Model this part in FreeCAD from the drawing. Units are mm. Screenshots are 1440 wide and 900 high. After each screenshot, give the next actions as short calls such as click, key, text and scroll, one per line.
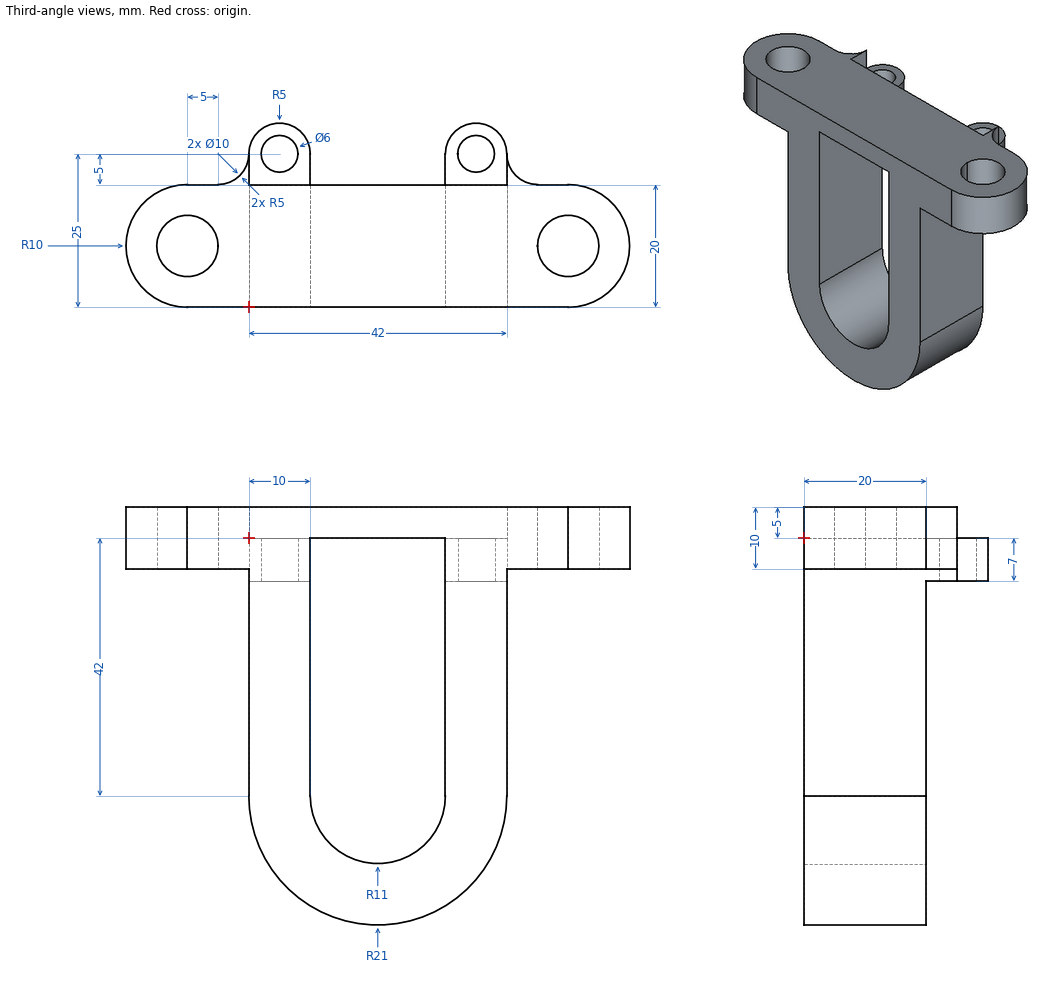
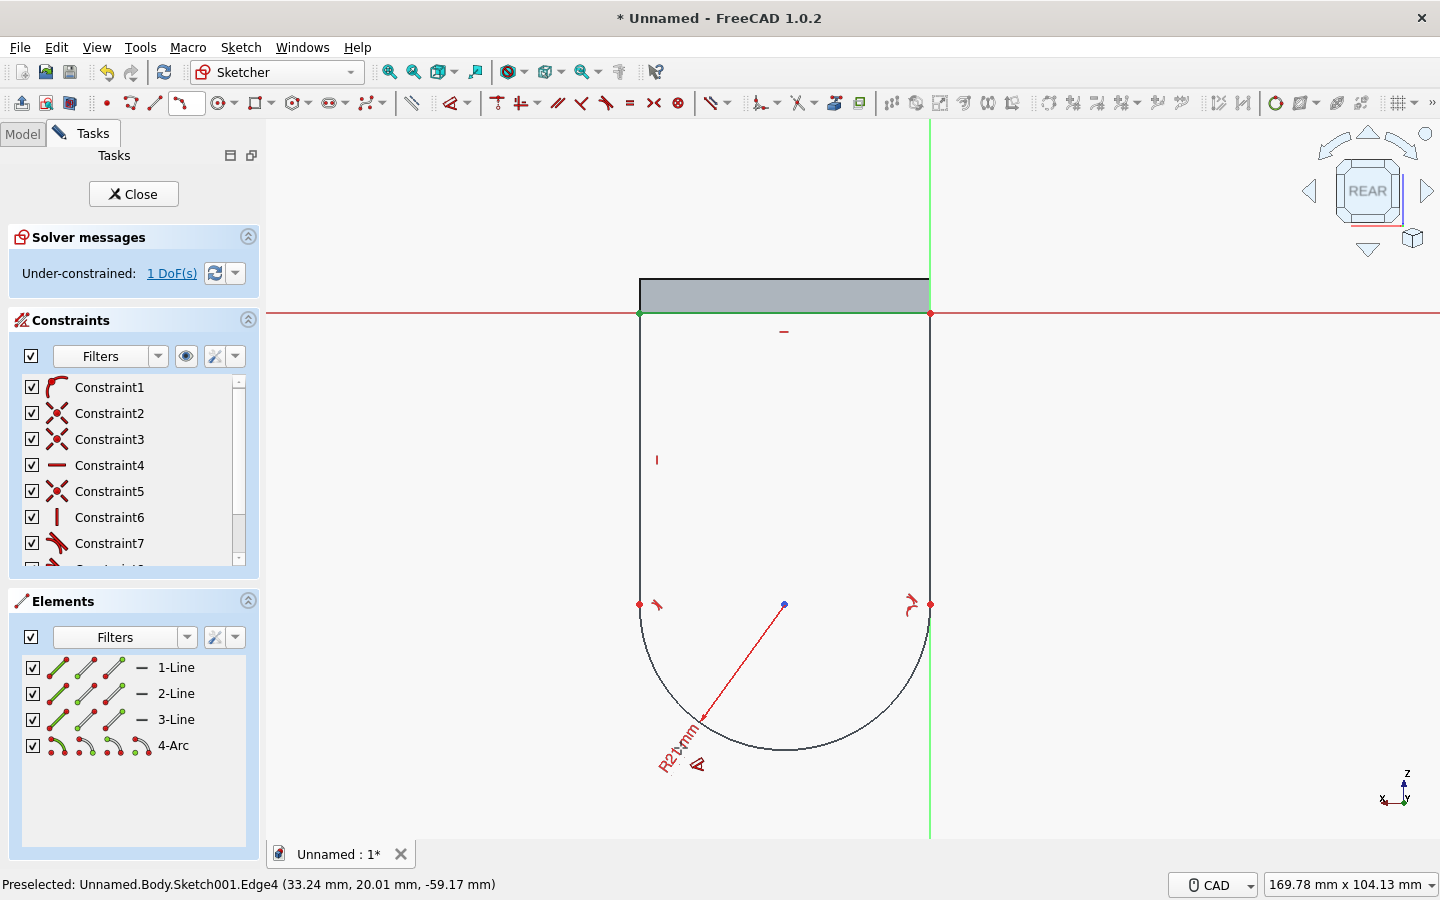
click(930, 517)
click(964, 459)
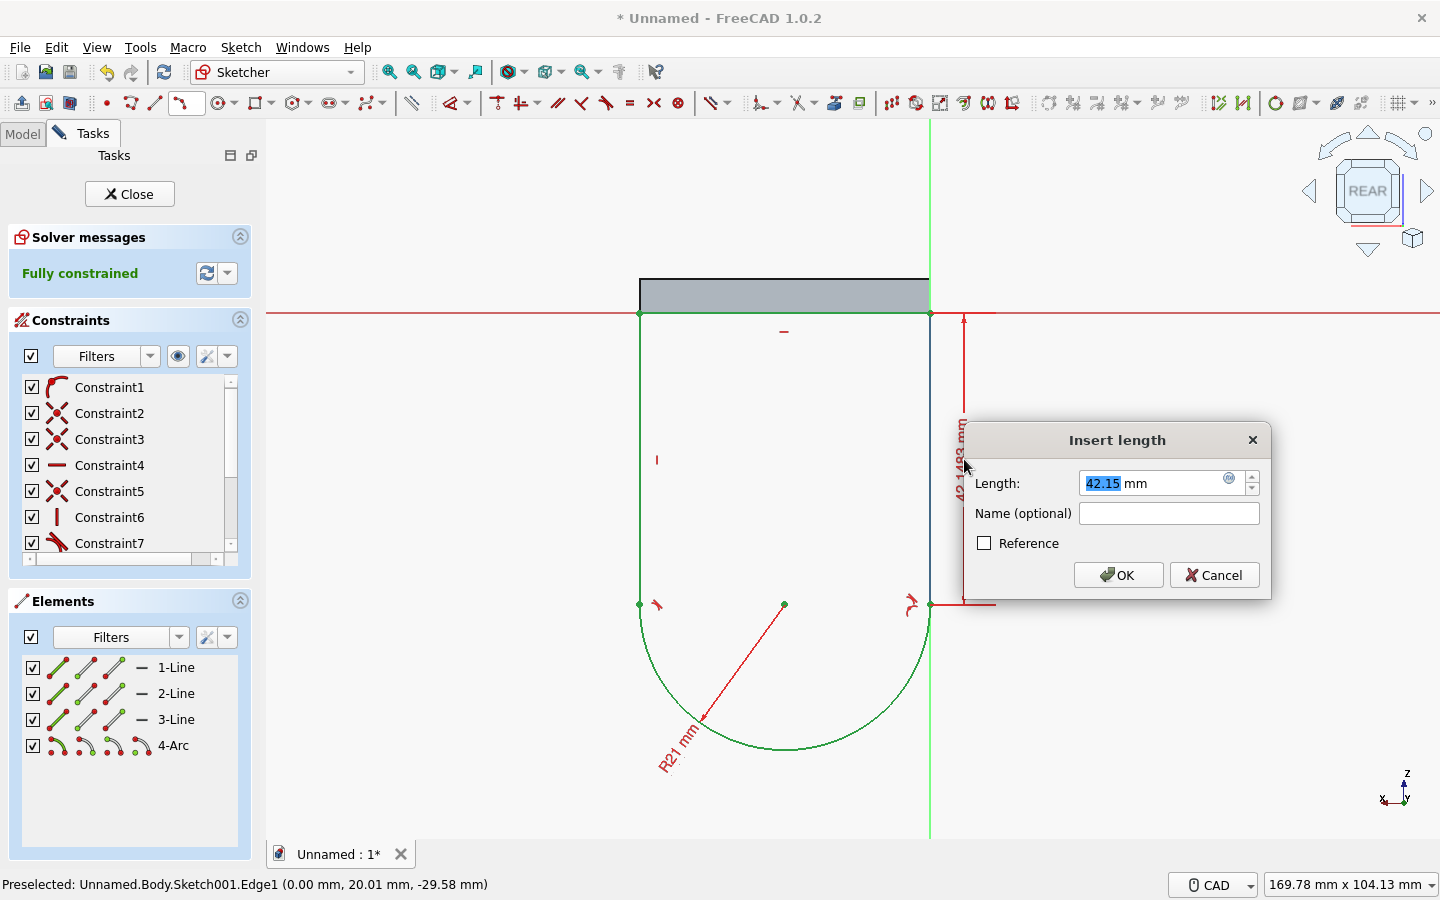
text(42)
key(Return)
key(Escape)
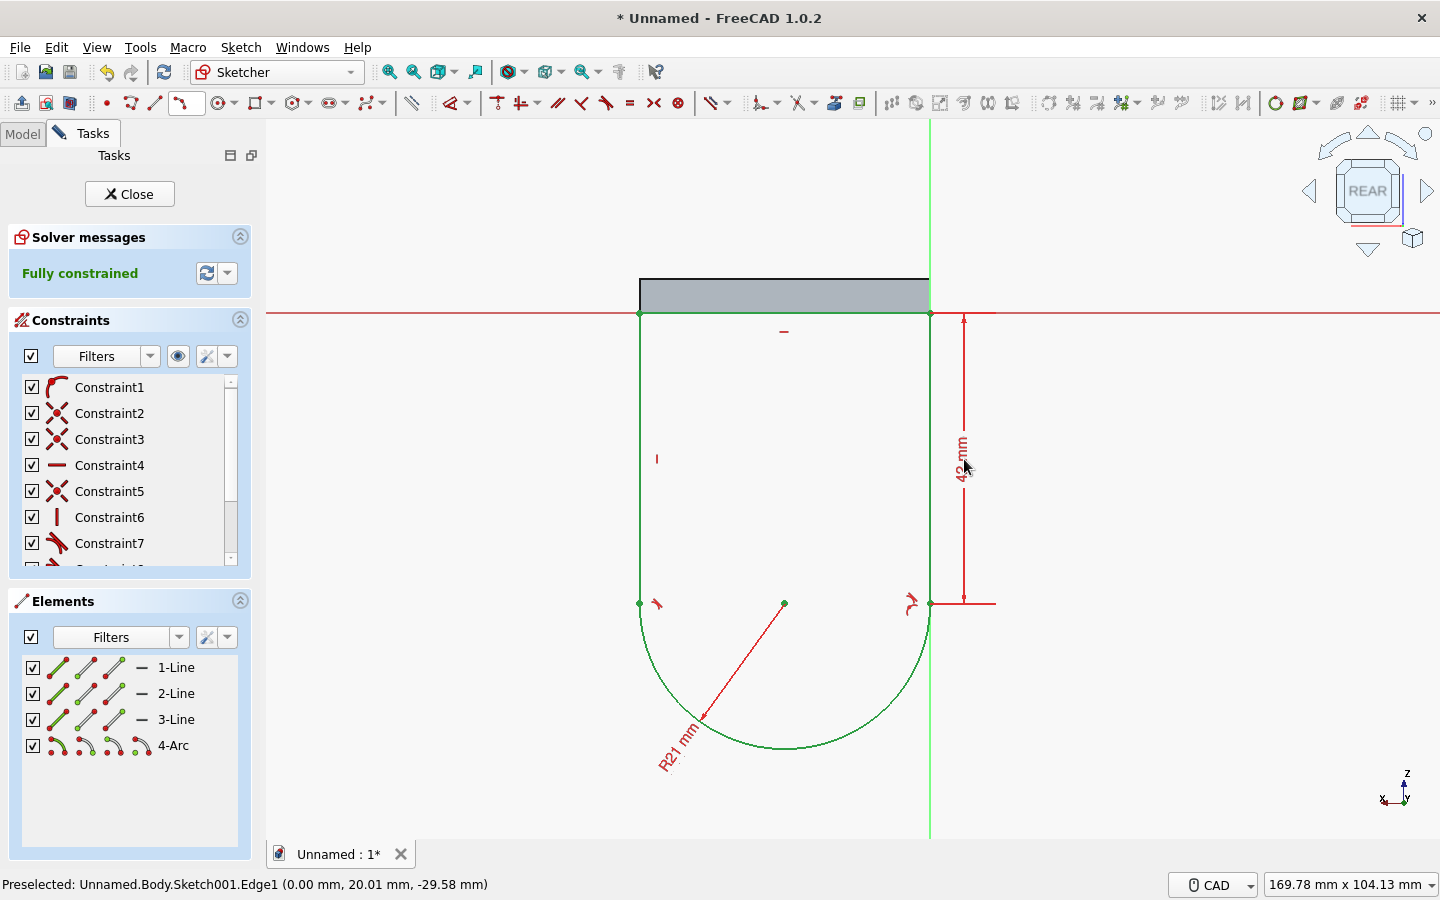
click(130, 194)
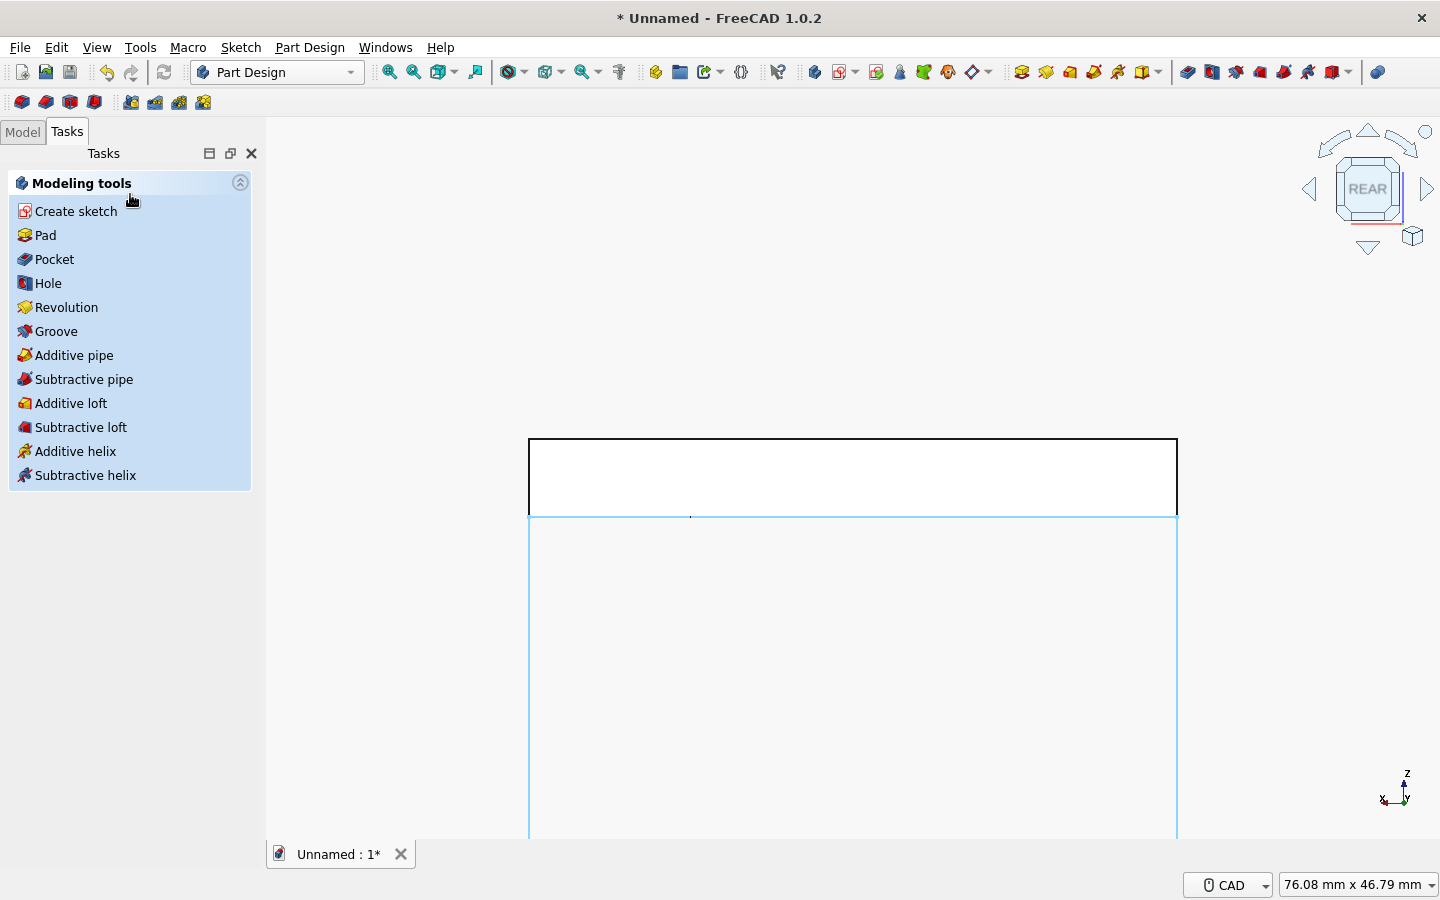
click(1022, 72)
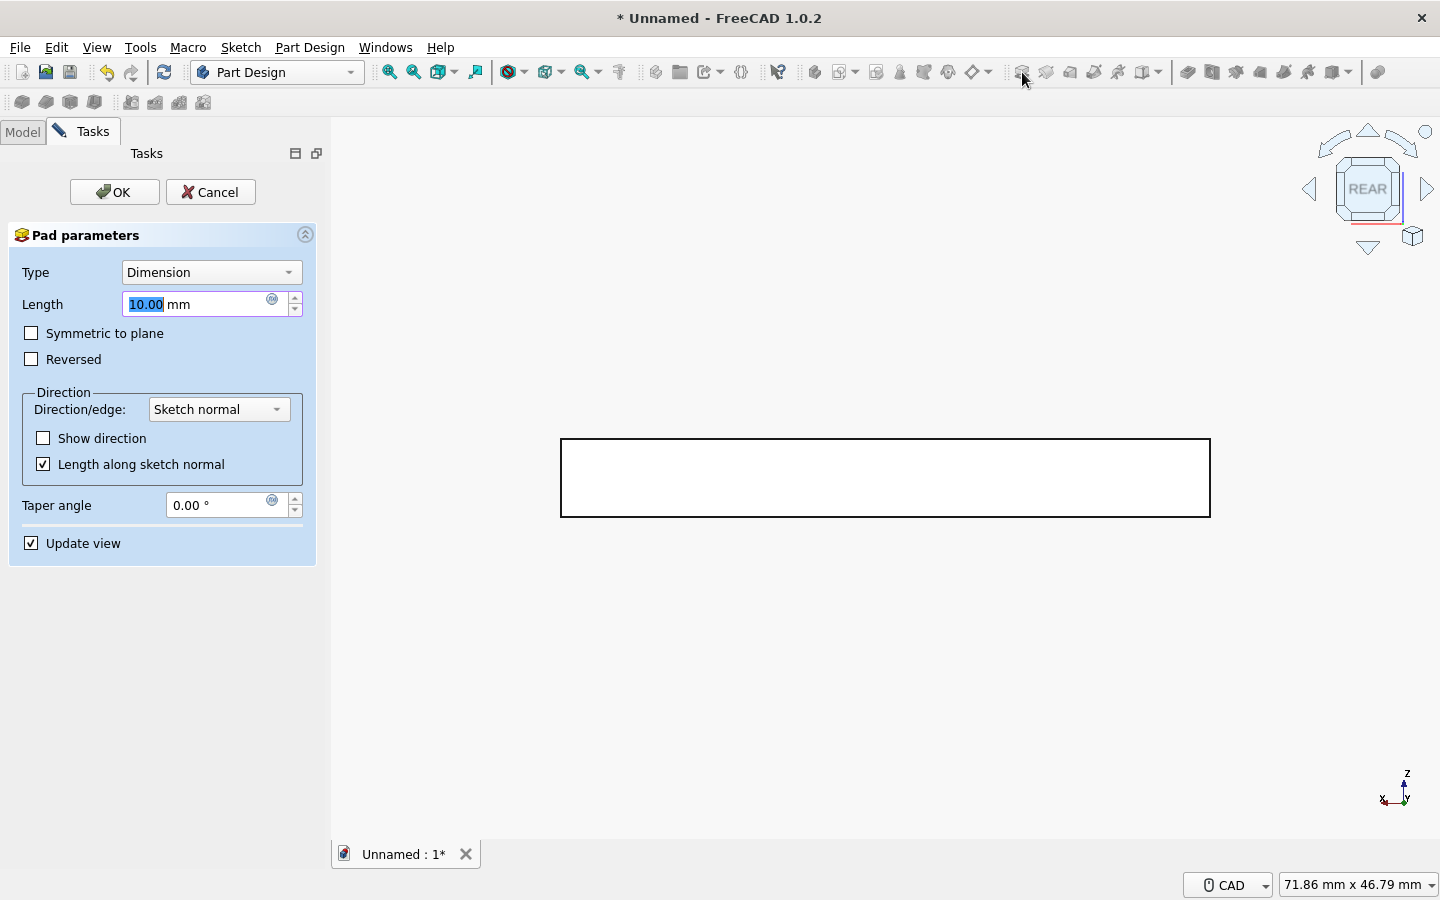
text(20)
key(Tab)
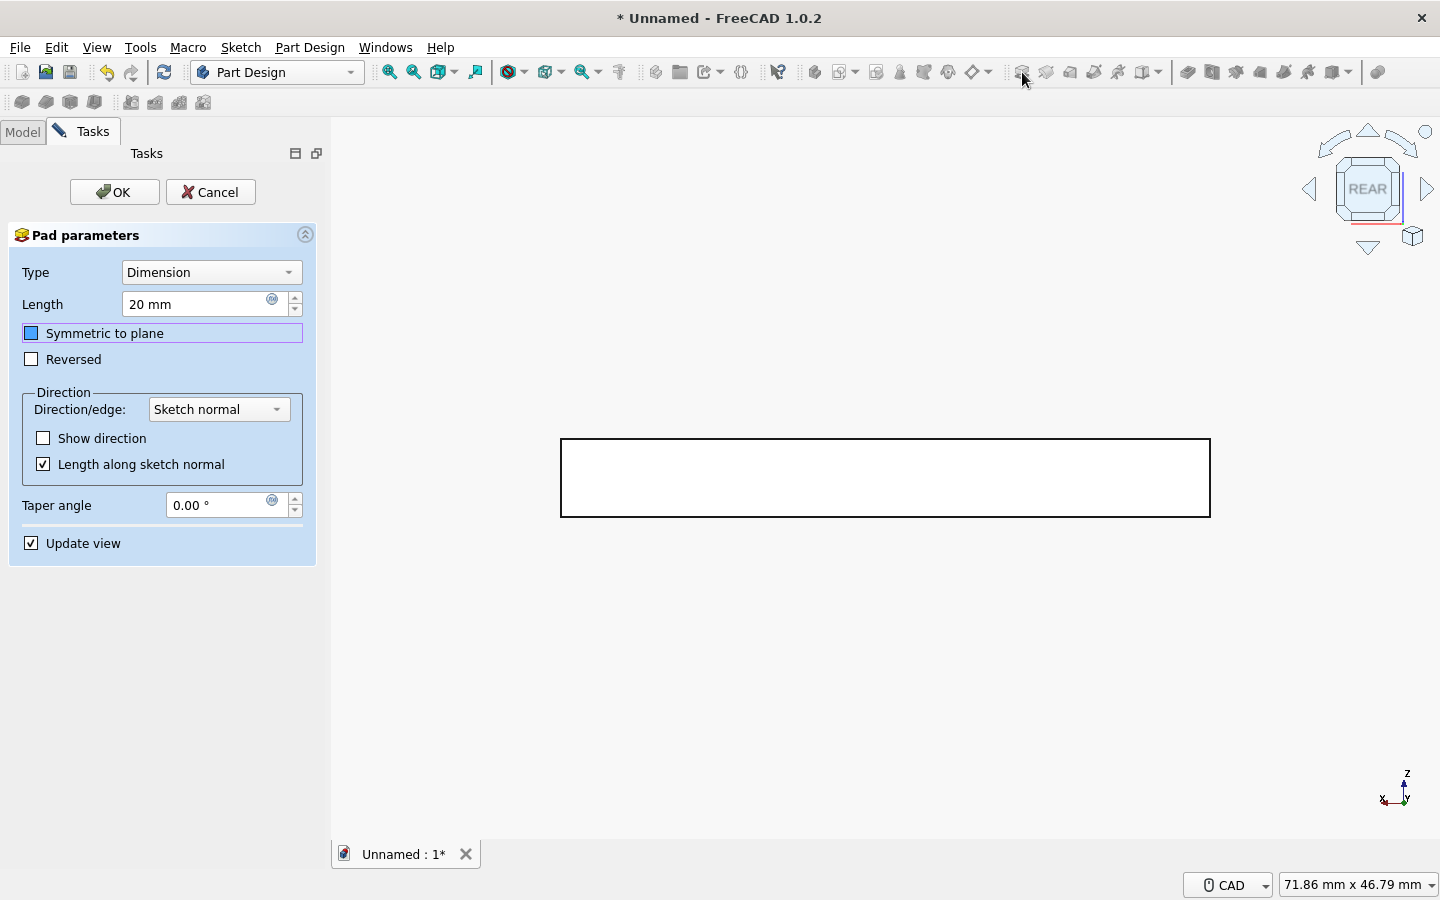
click(30, 359)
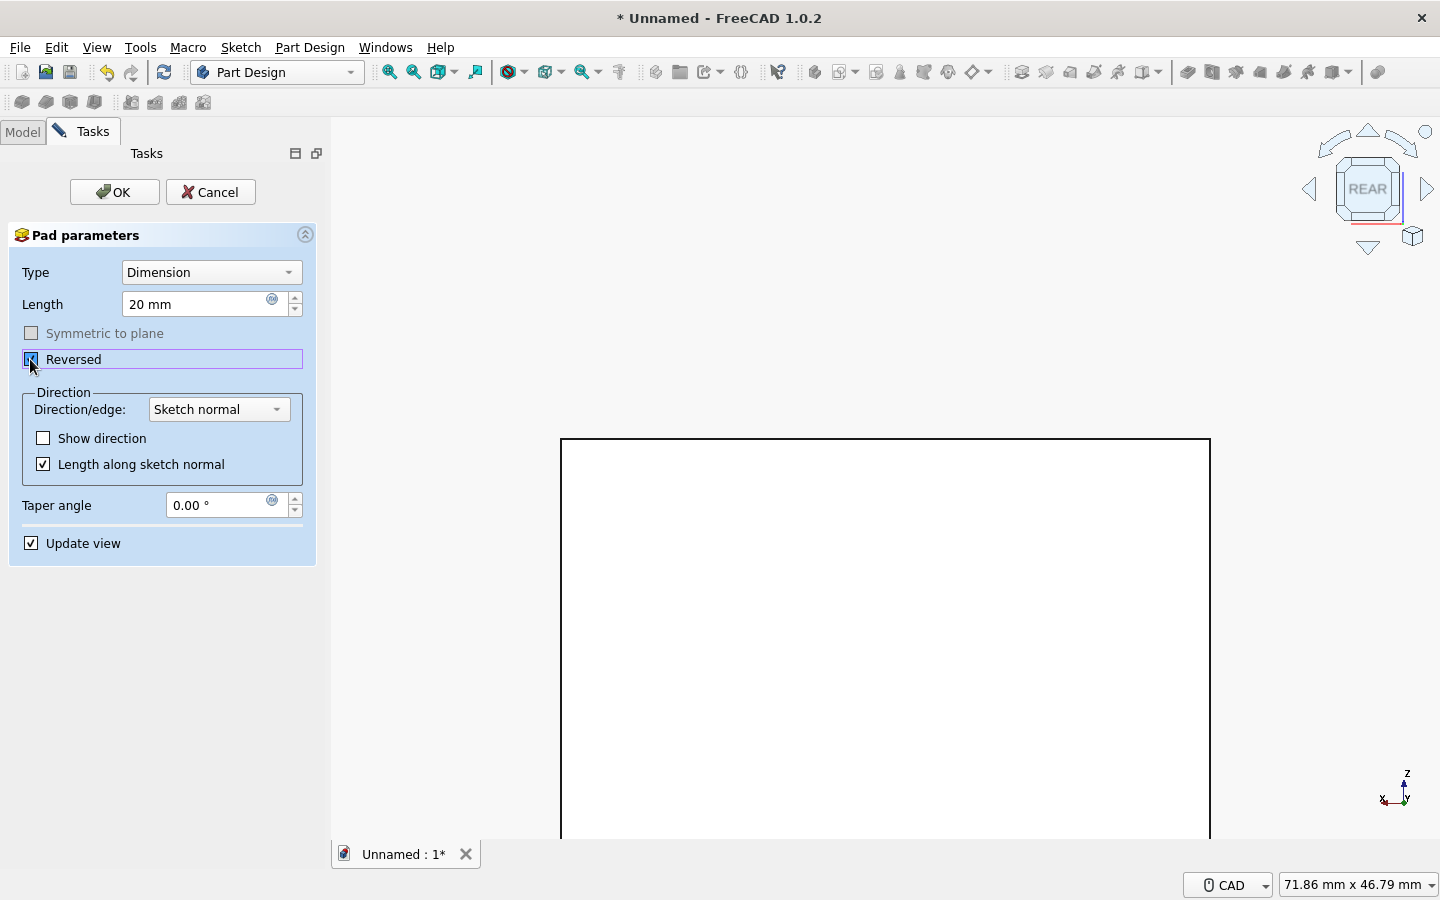
click(115, 192)